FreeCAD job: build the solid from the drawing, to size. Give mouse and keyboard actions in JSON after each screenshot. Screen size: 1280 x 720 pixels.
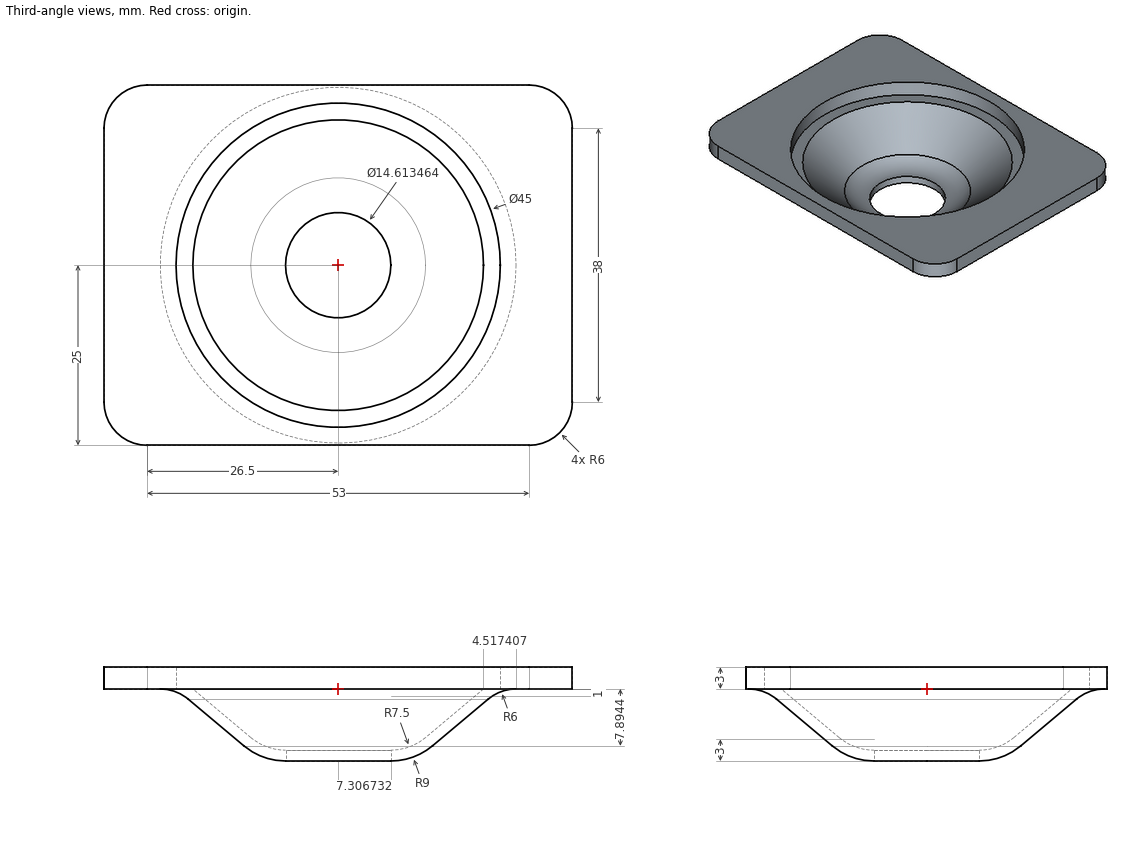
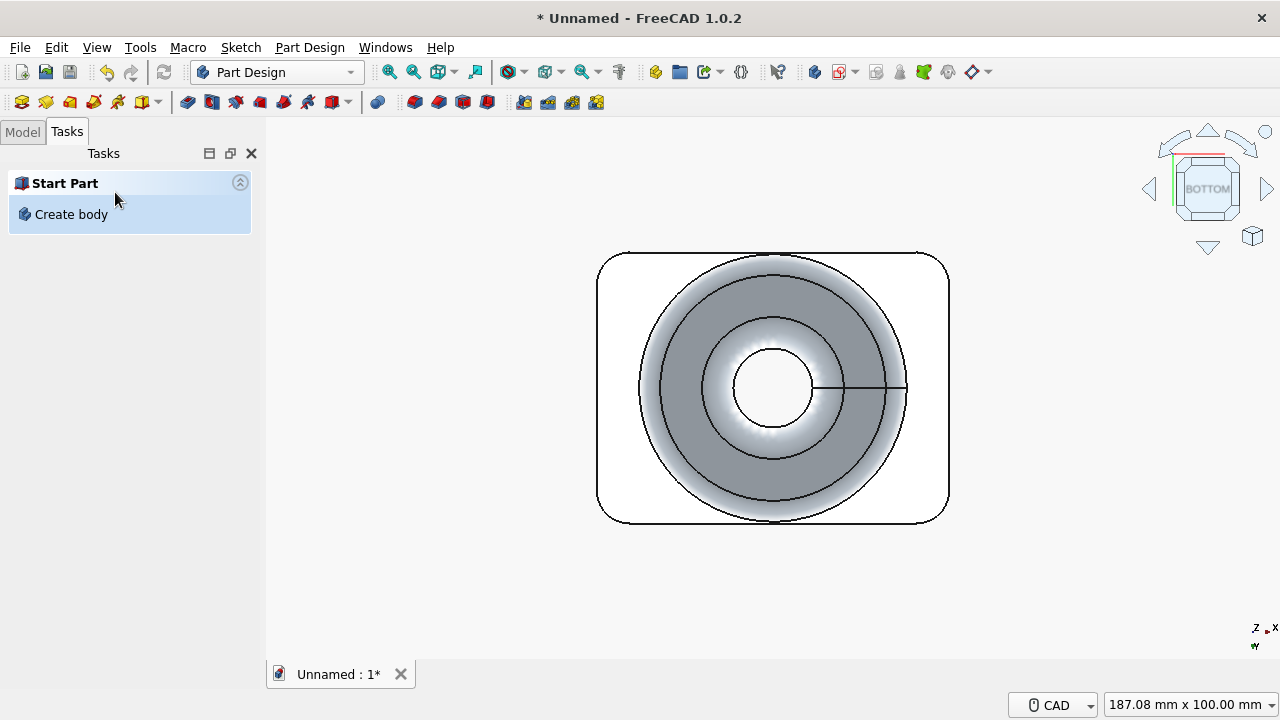
{"action": "key", "text": "0"}